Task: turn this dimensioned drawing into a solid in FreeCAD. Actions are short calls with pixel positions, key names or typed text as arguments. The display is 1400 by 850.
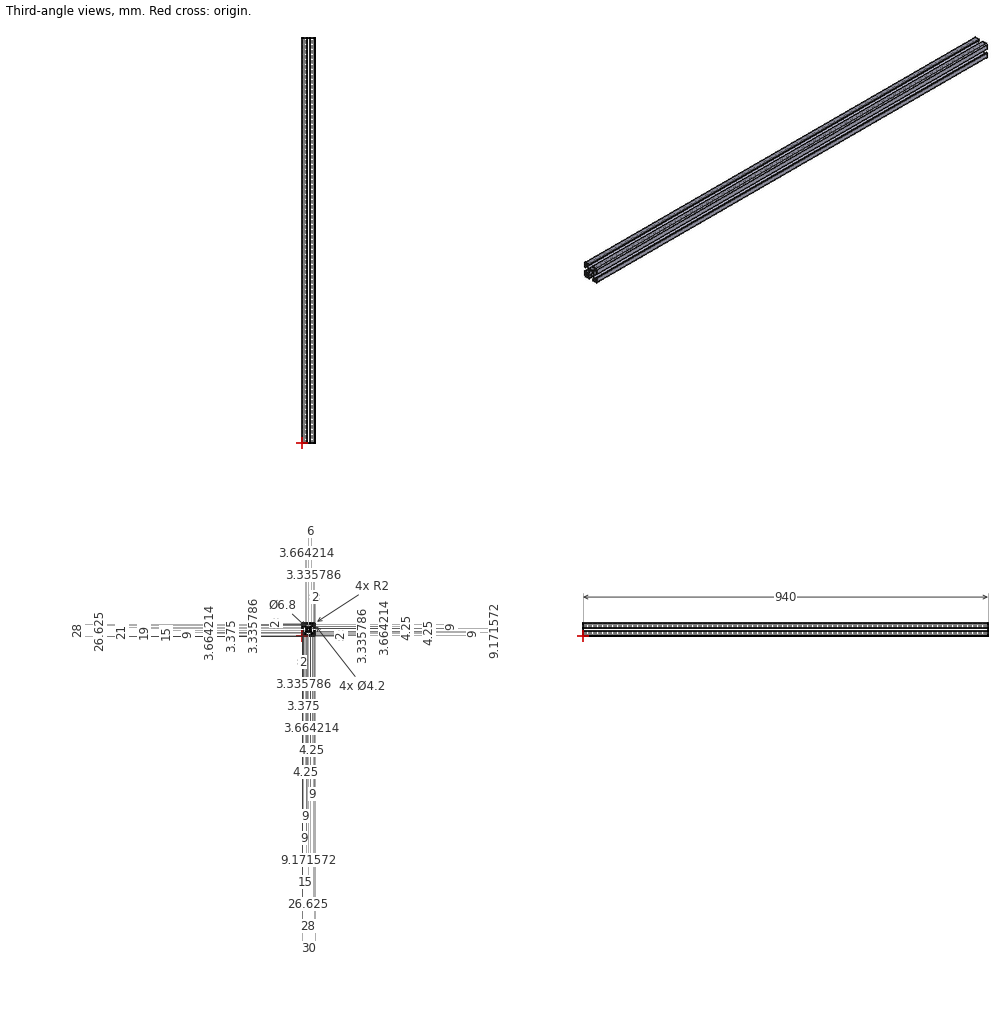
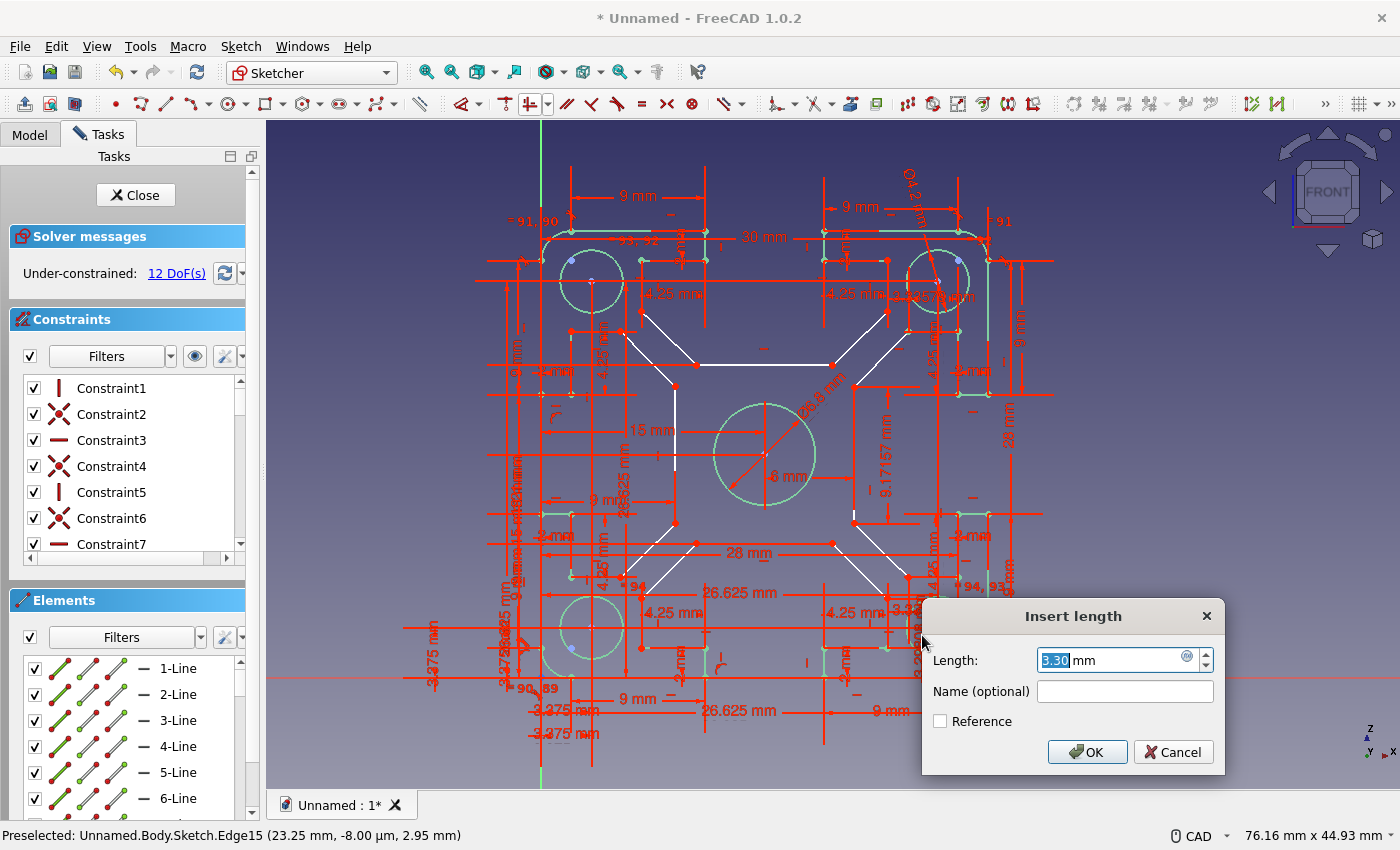
text(3.335786)
key(Return)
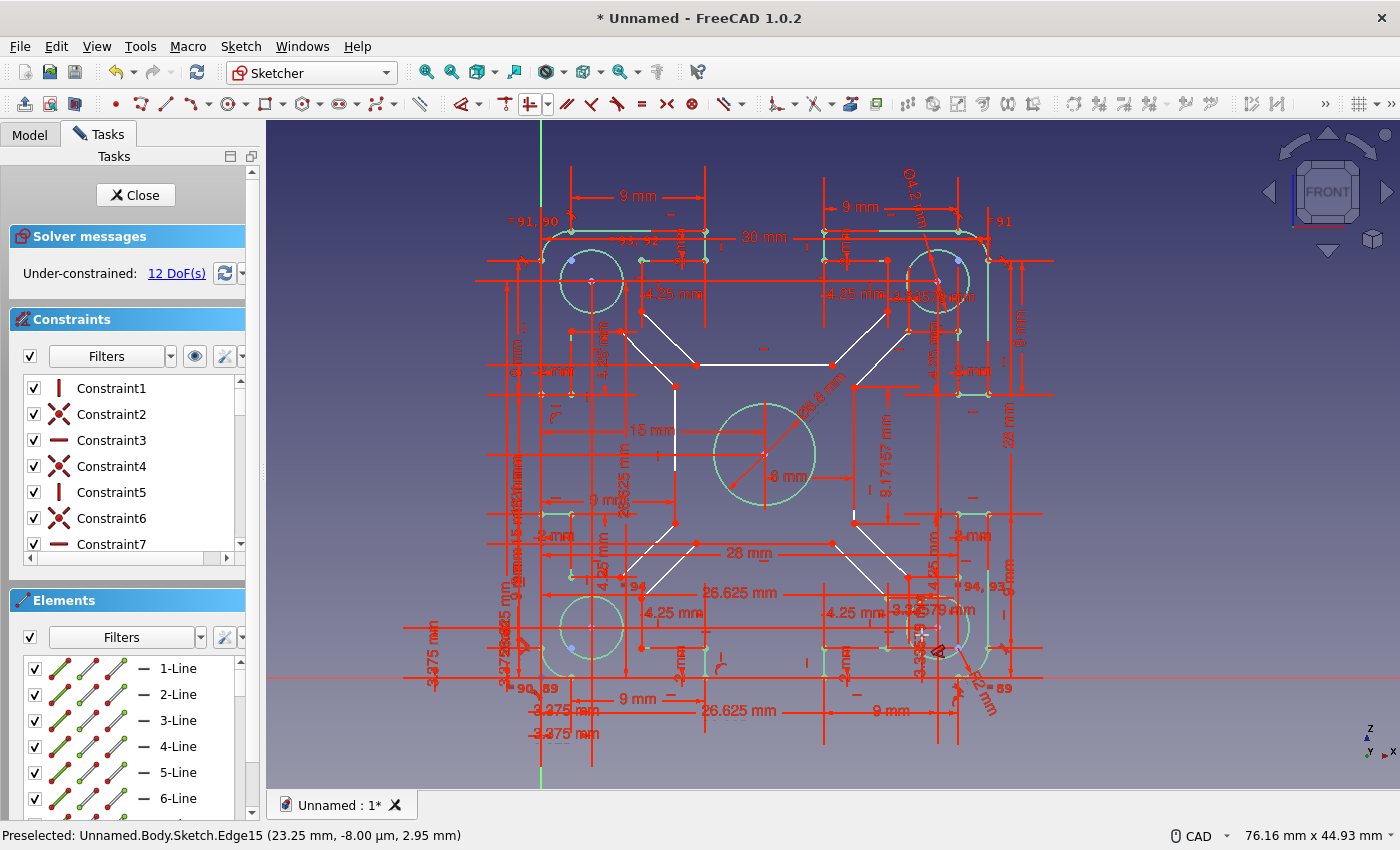
click(792, 544)
click(813, 578)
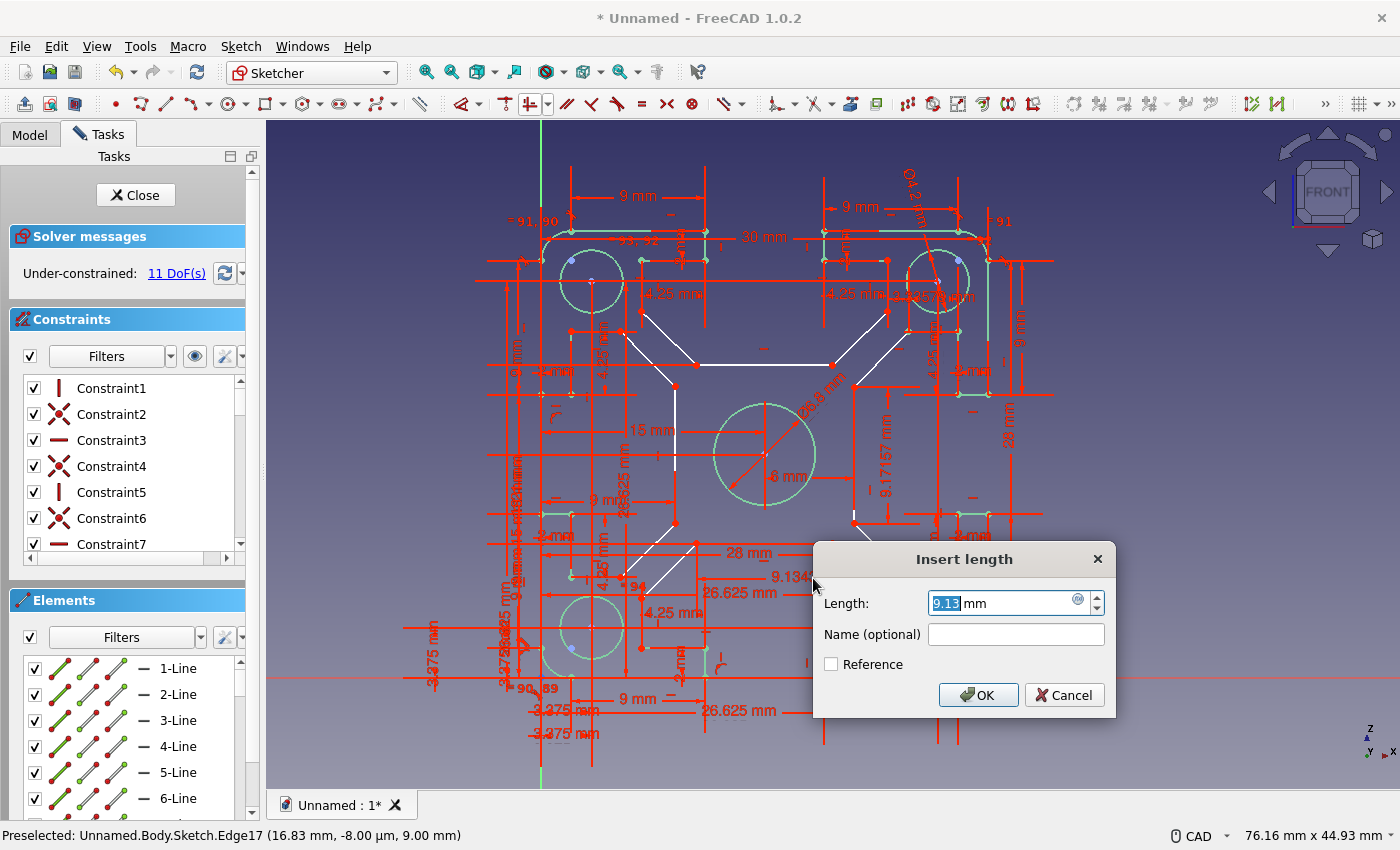
text(9.171572)
key(Return)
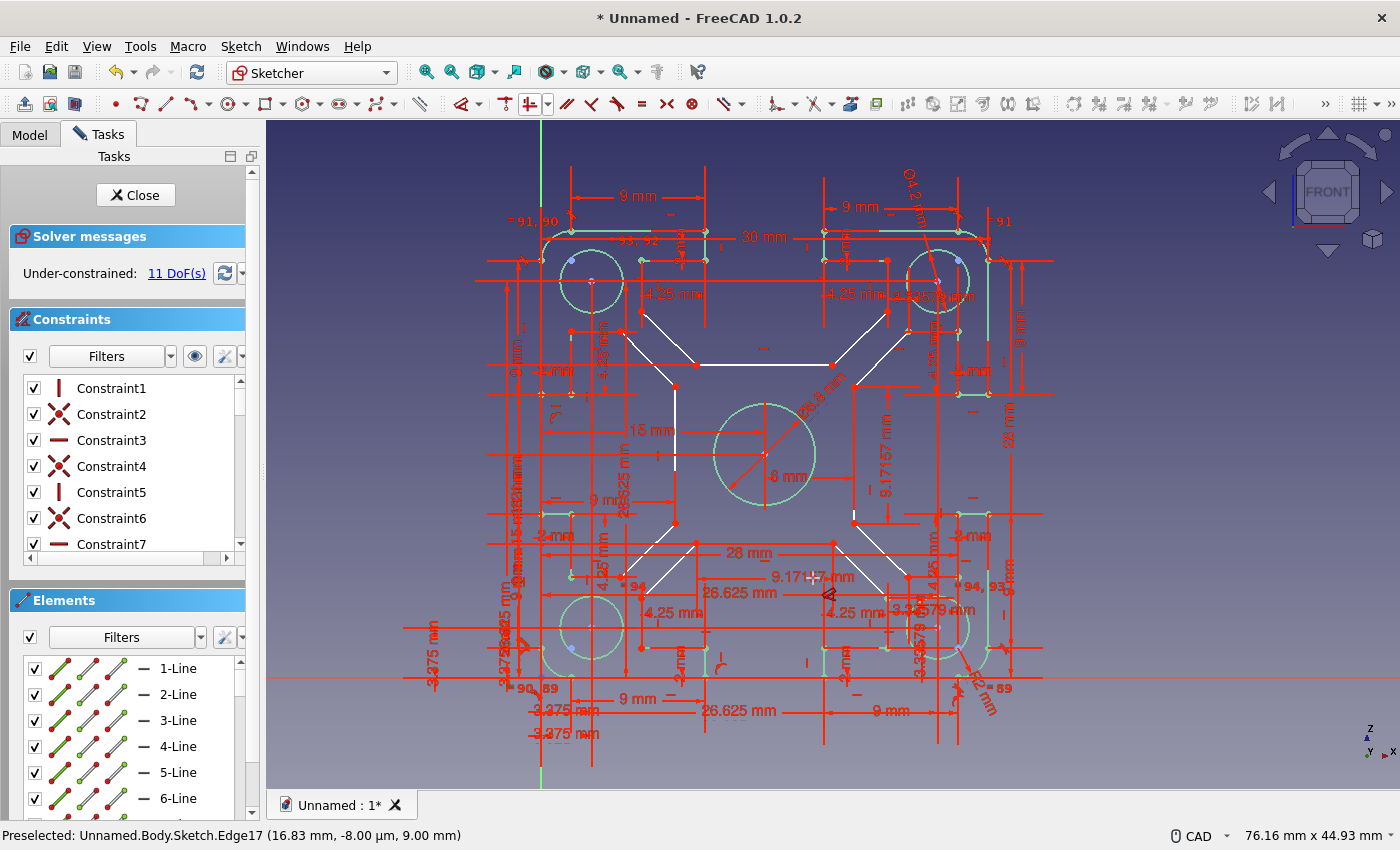
click(642, 614)
click(608, 635)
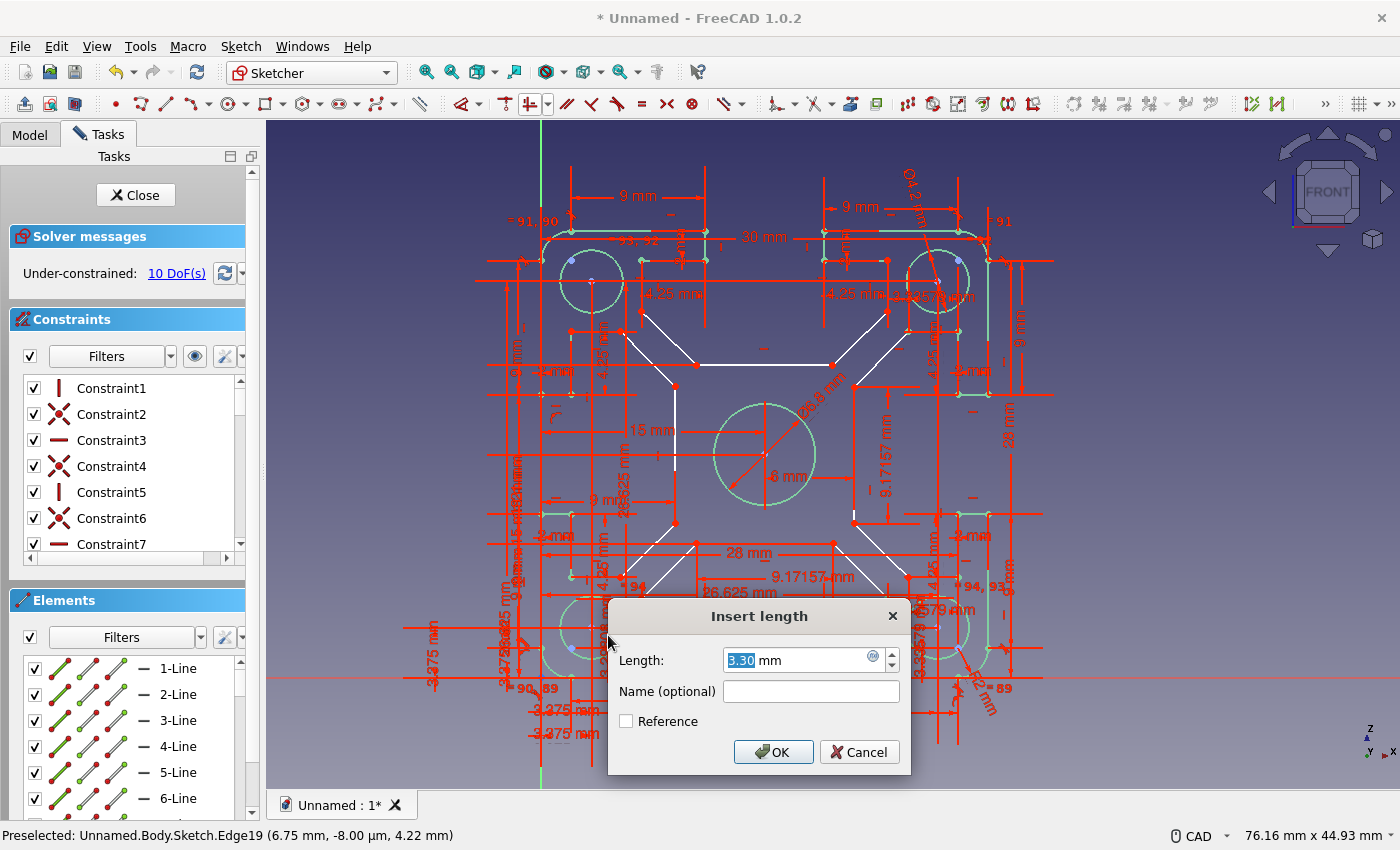
text(3.335786)
key(Return)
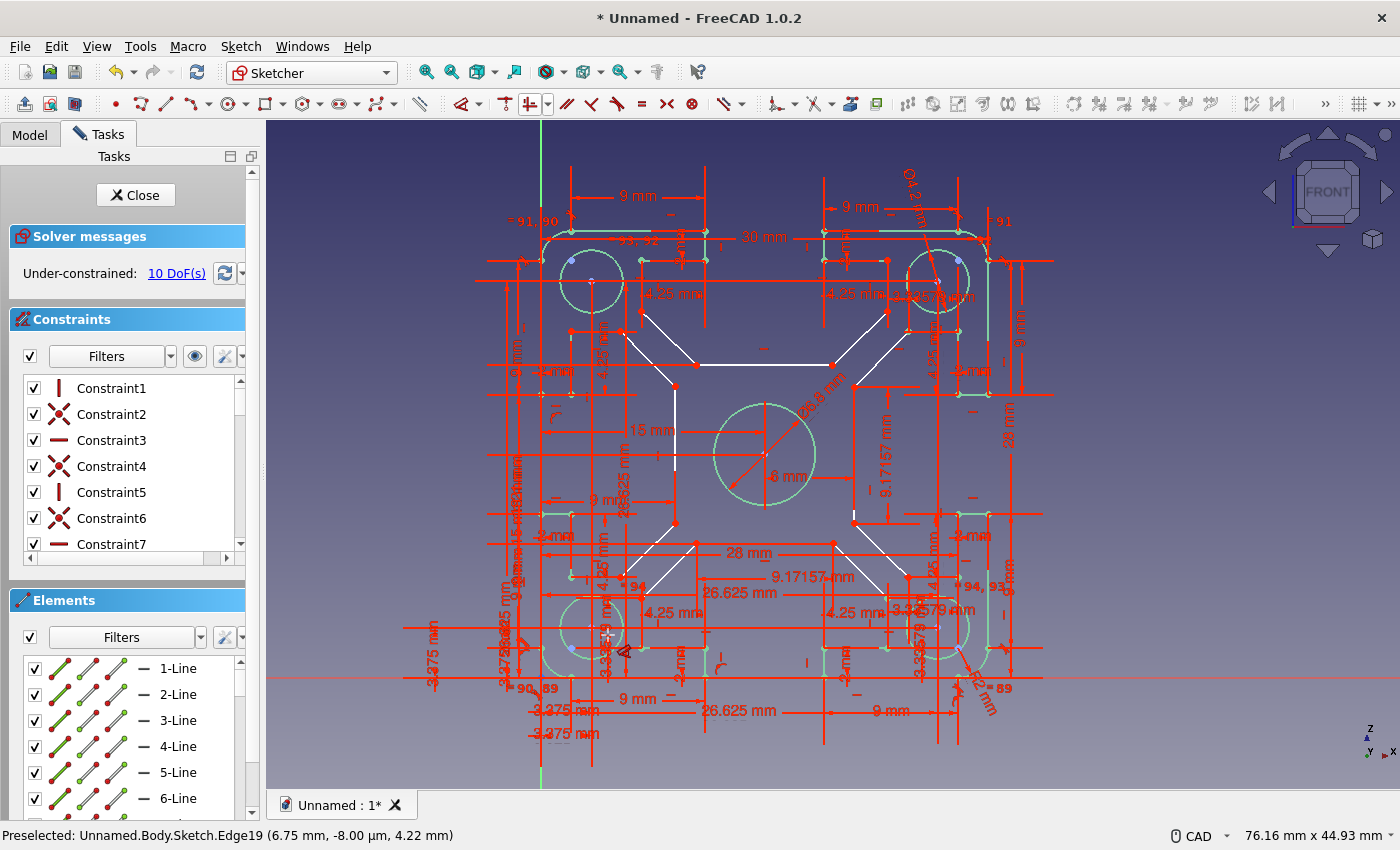
click(586, 577)
click(596, 611)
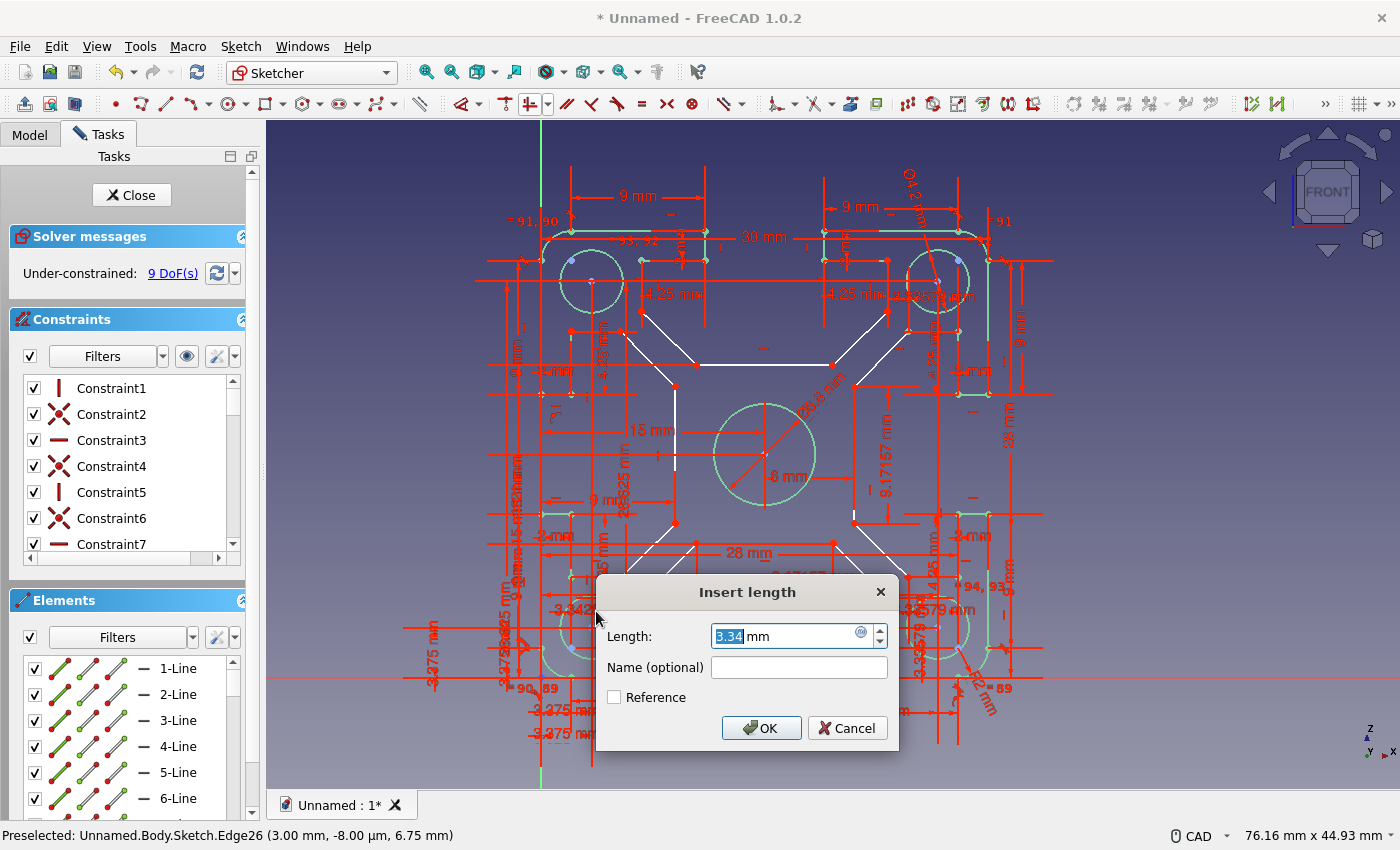
text(3.335786)
key(Return)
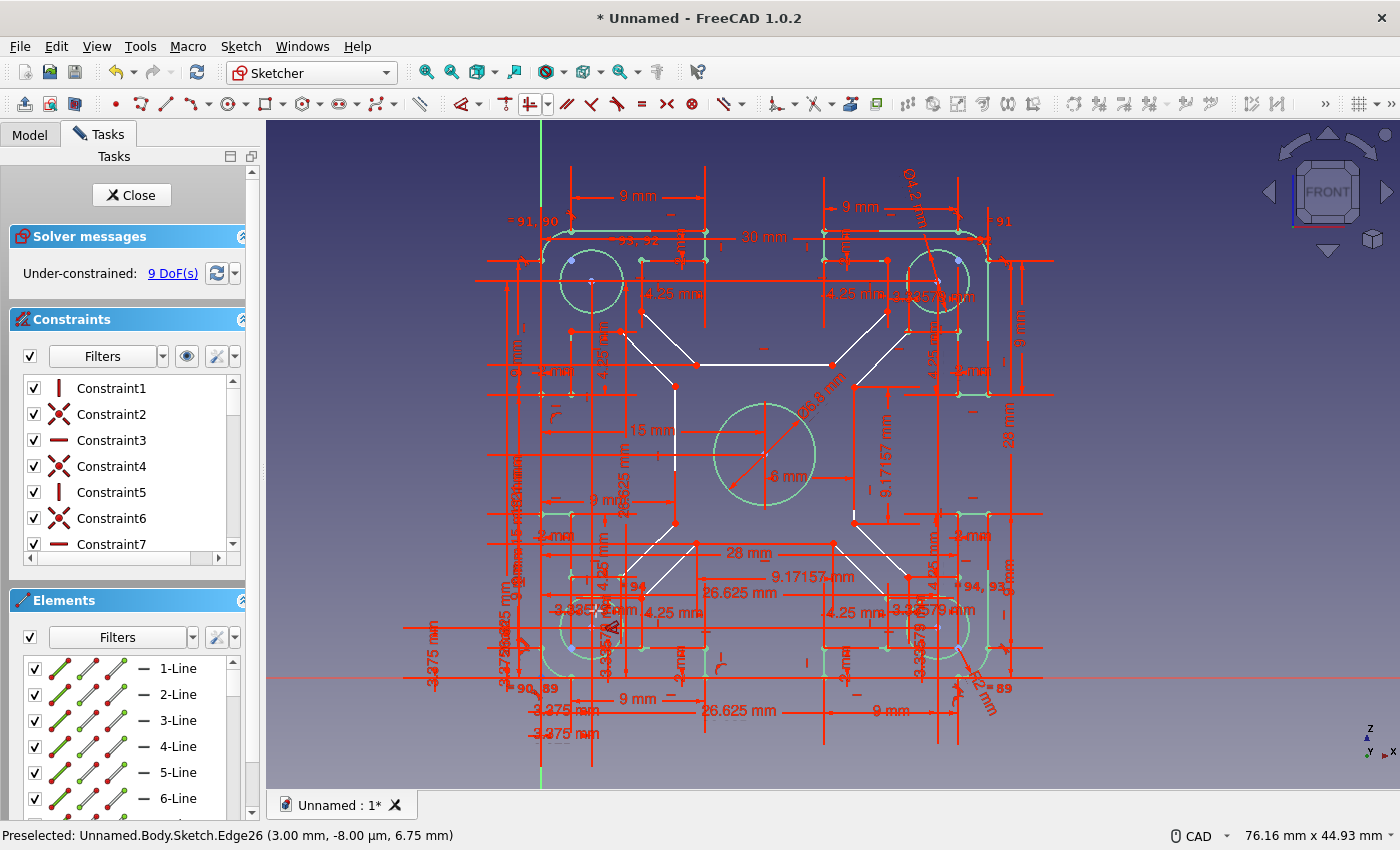
click(675, 483)
click(641, 455)